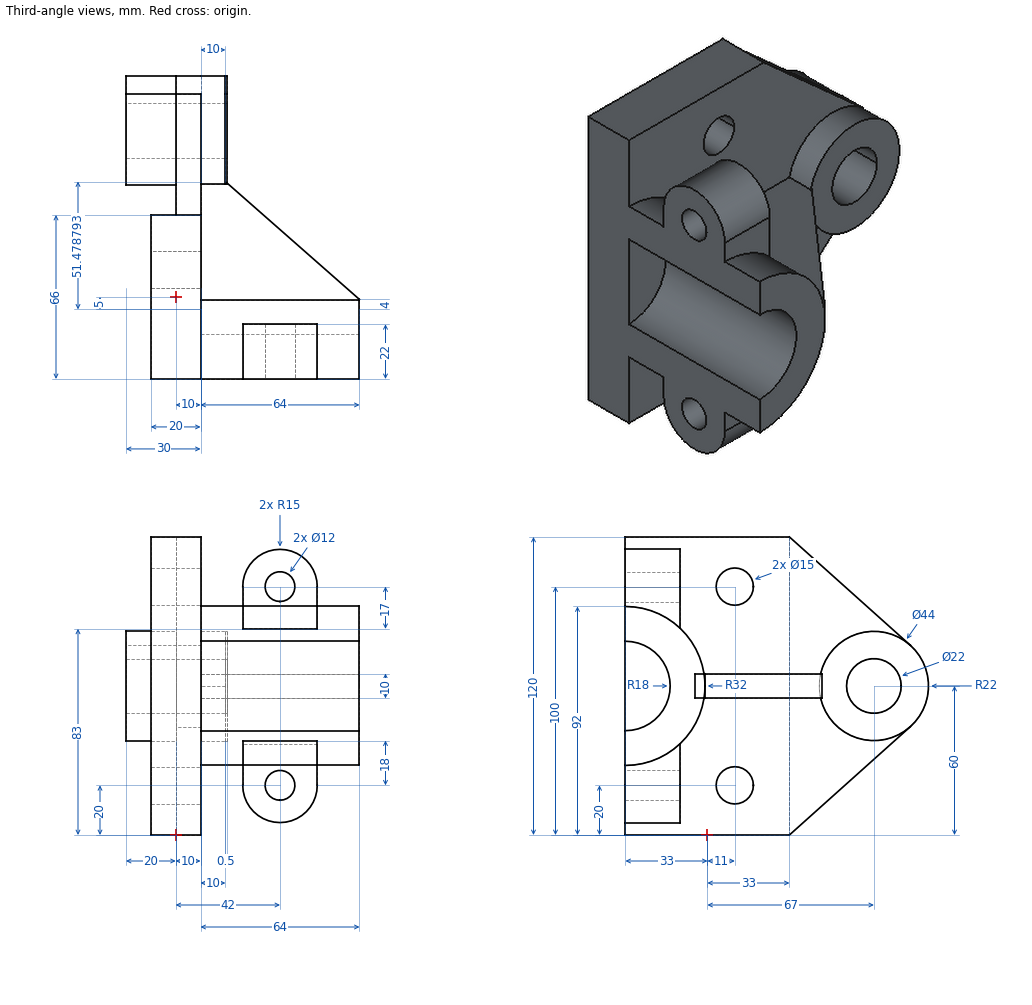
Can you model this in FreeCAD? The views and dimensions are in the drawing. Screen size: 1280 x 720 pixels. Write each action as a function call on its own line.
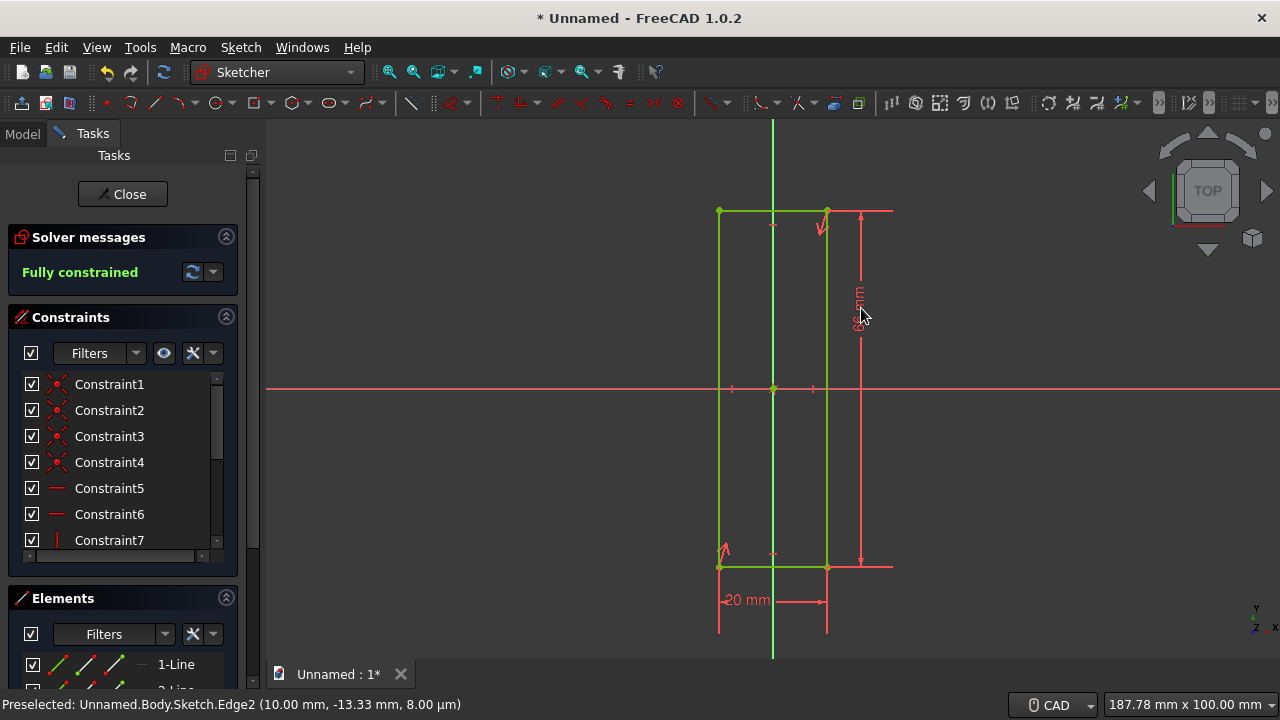
click(123, 194)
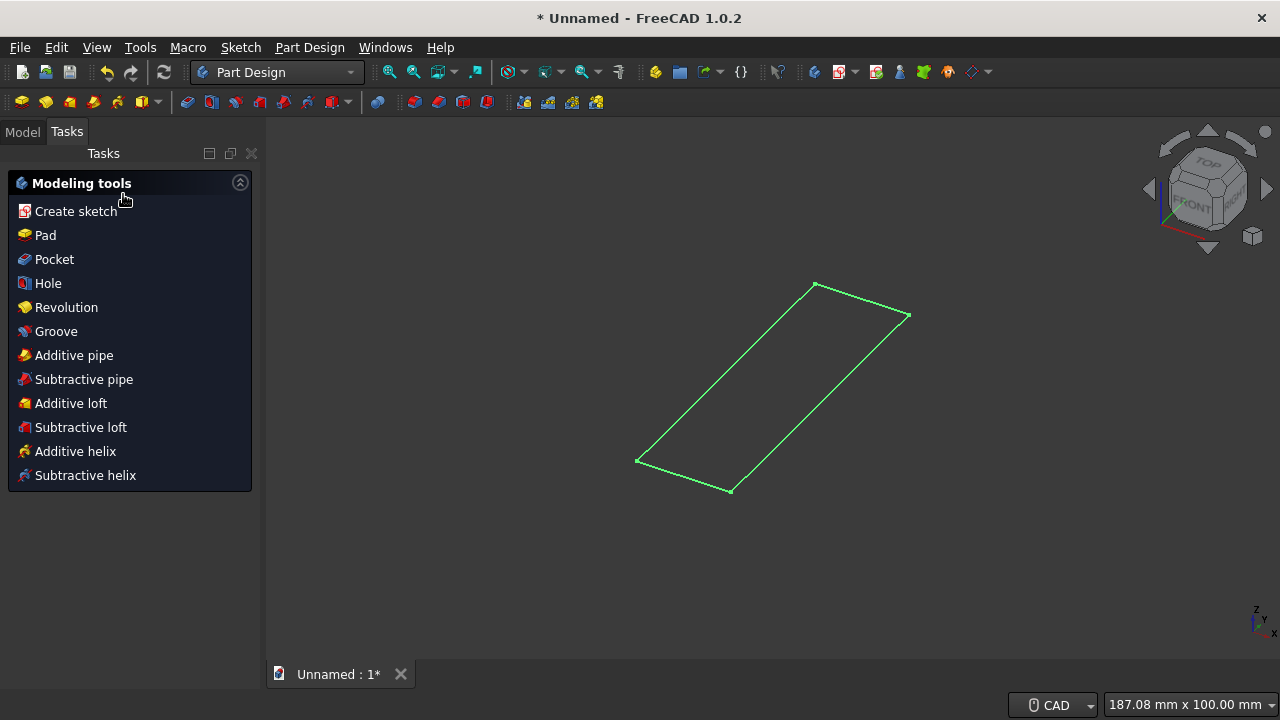
click(22, 102)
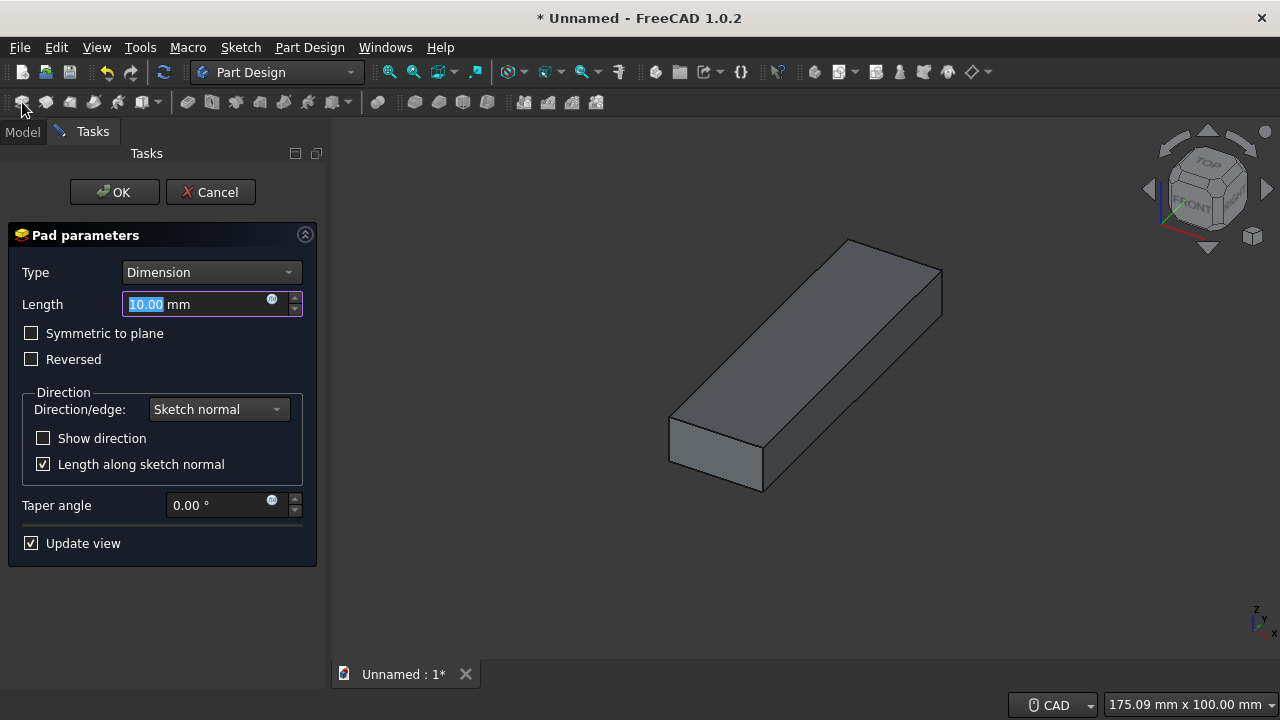
text(120)
key(Tab)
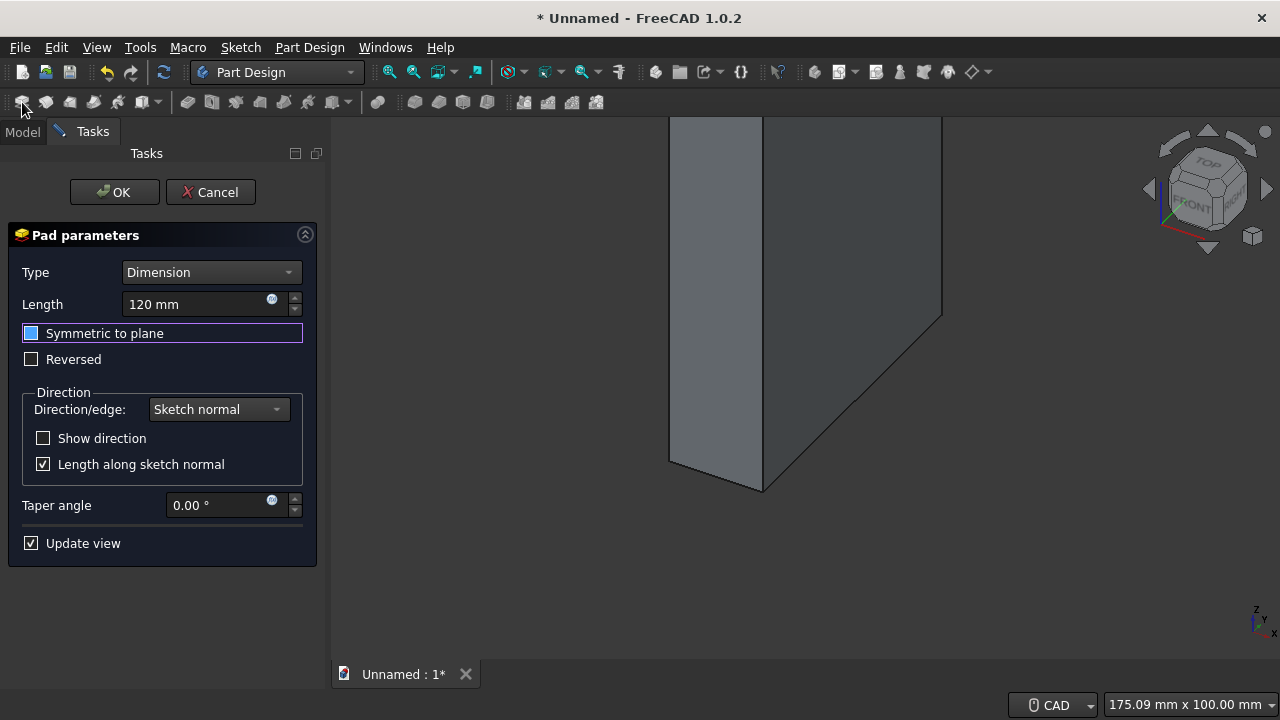
click(115, 192)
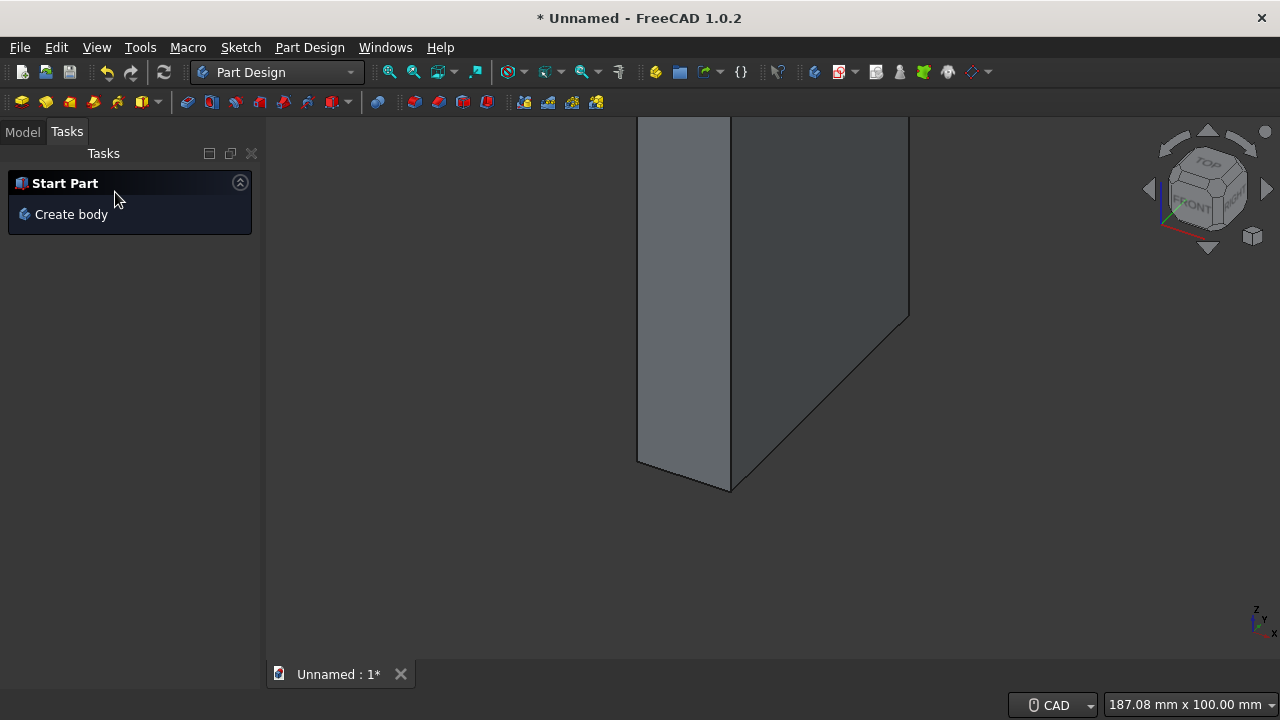
click(390, 72)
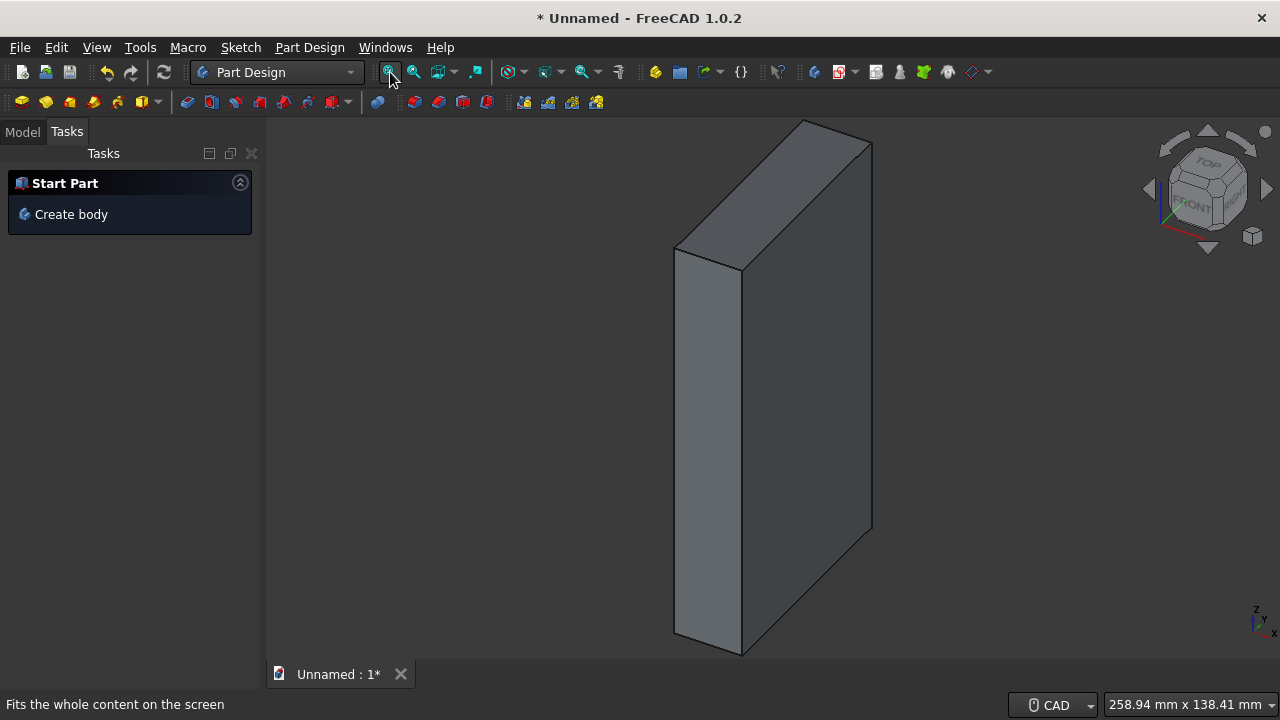
click(807, 343)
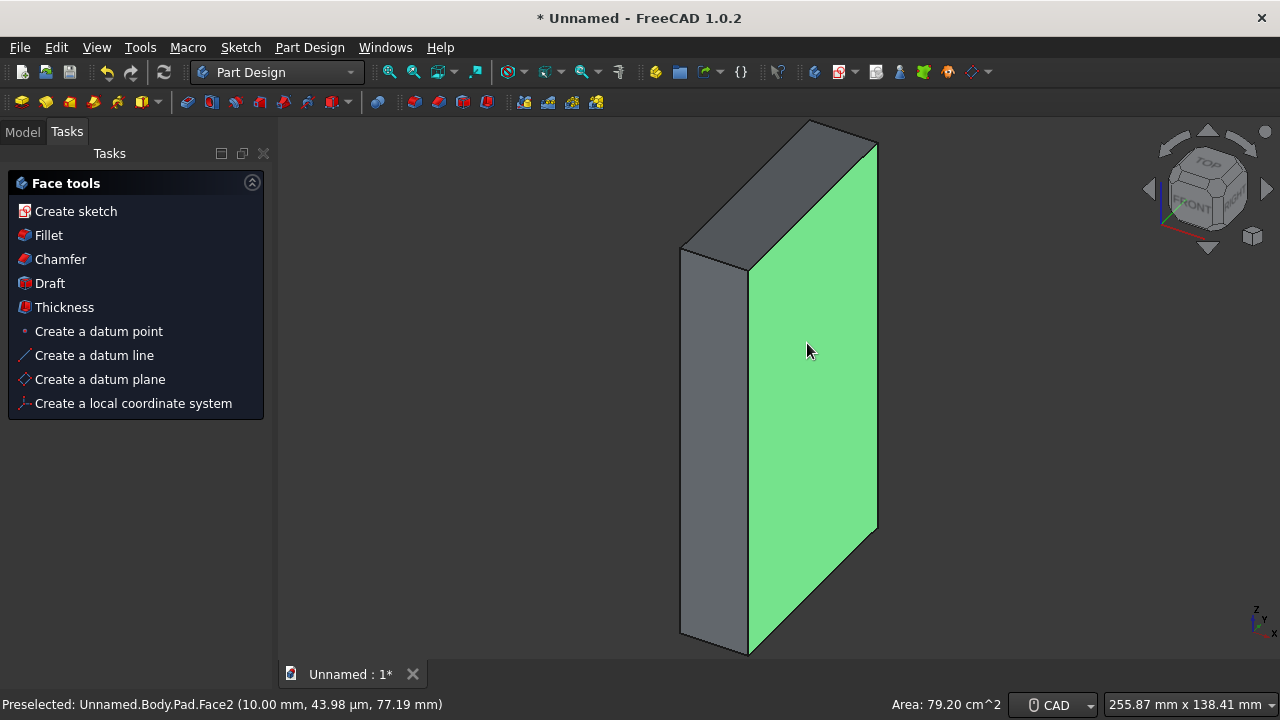
click(840, 72)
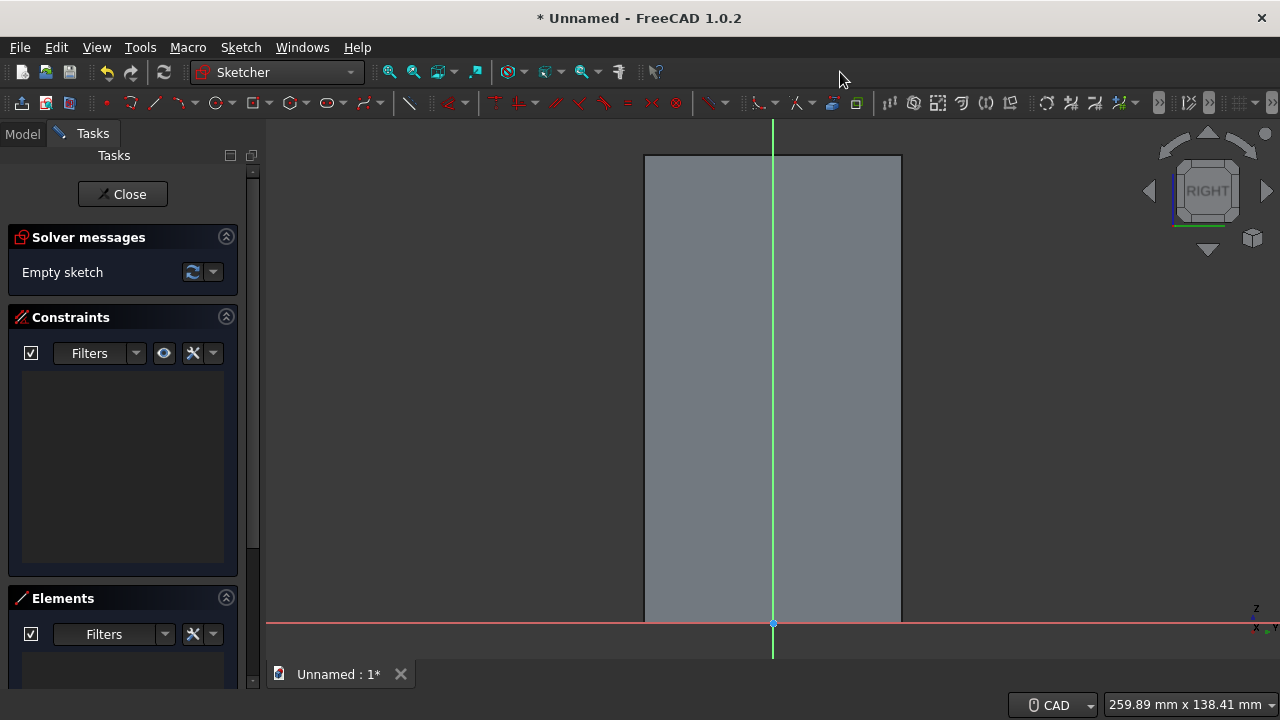
scroll(294, 389, down, 2)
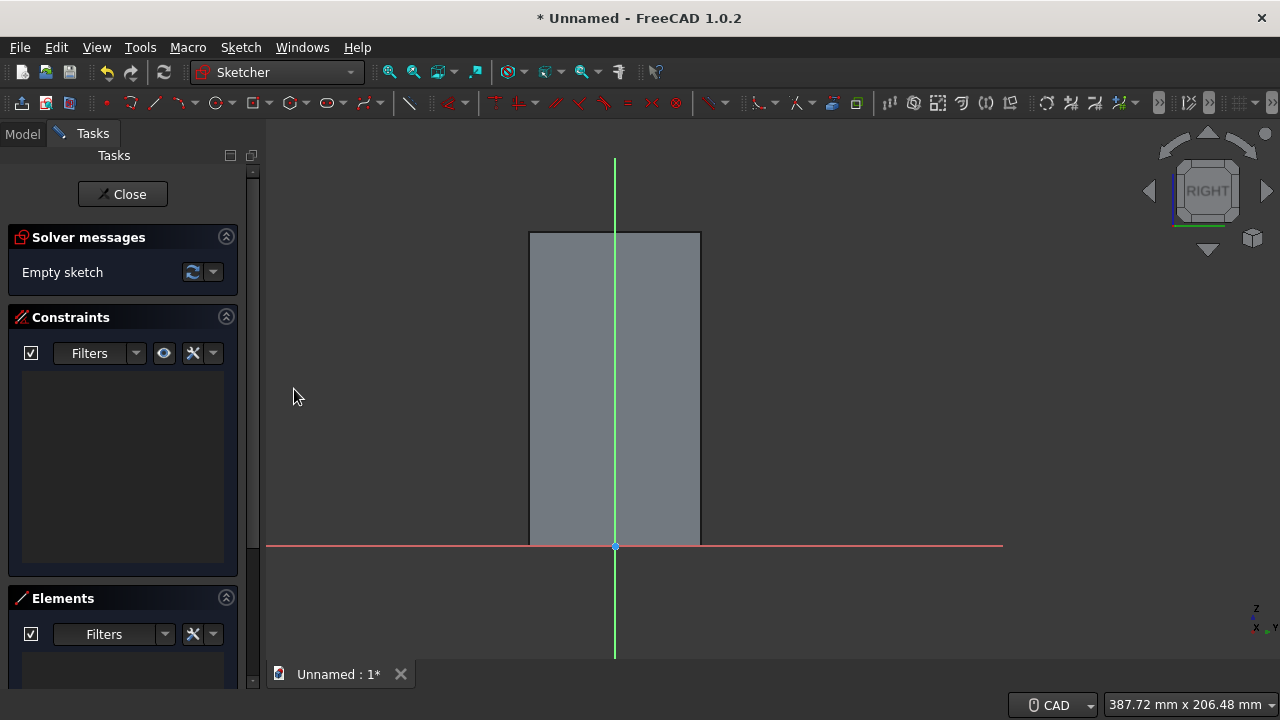
click(132, 104)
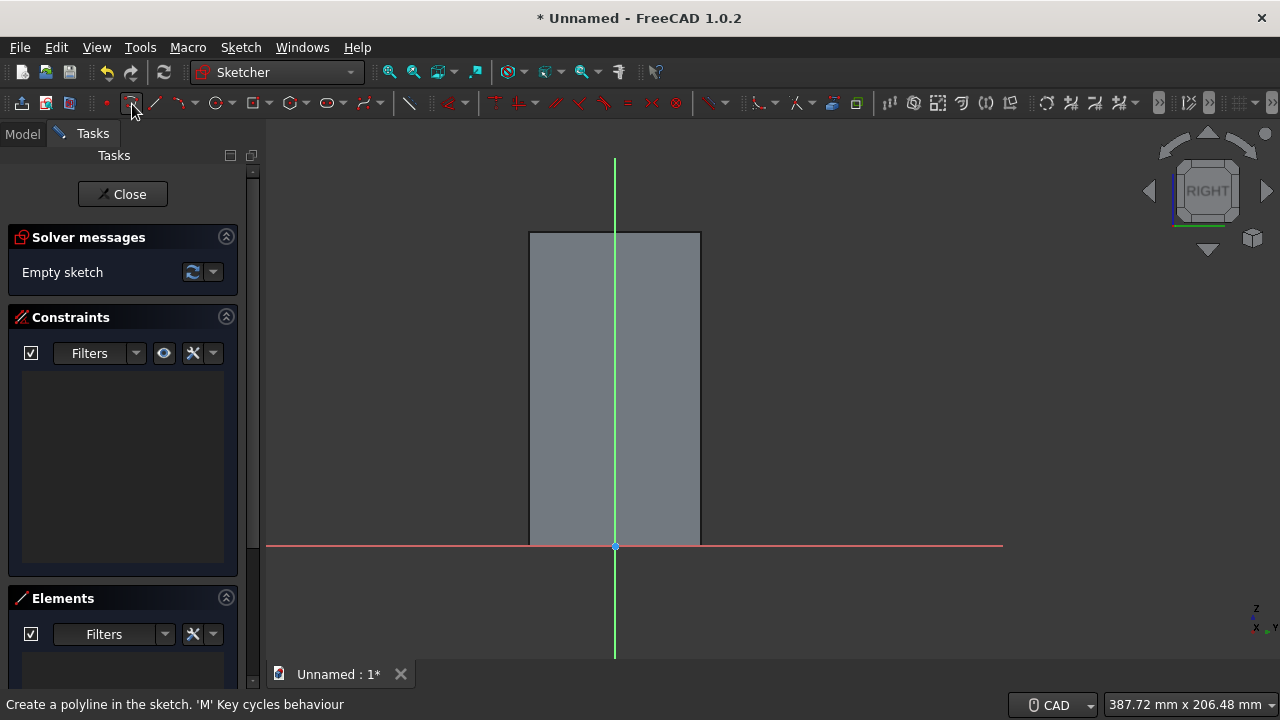
click(829, 346)
click(701, 232)
click(701, 546)
click(829, 432)
right_click(829, 432)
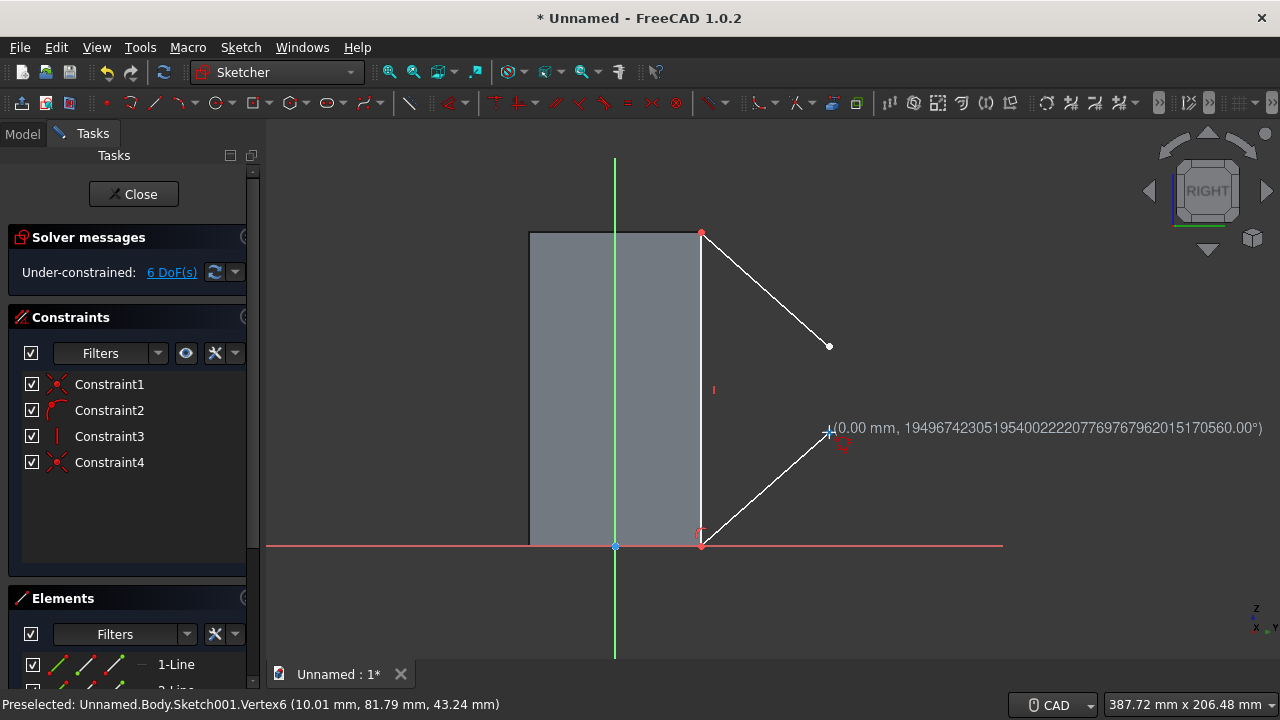
click(180, 104)